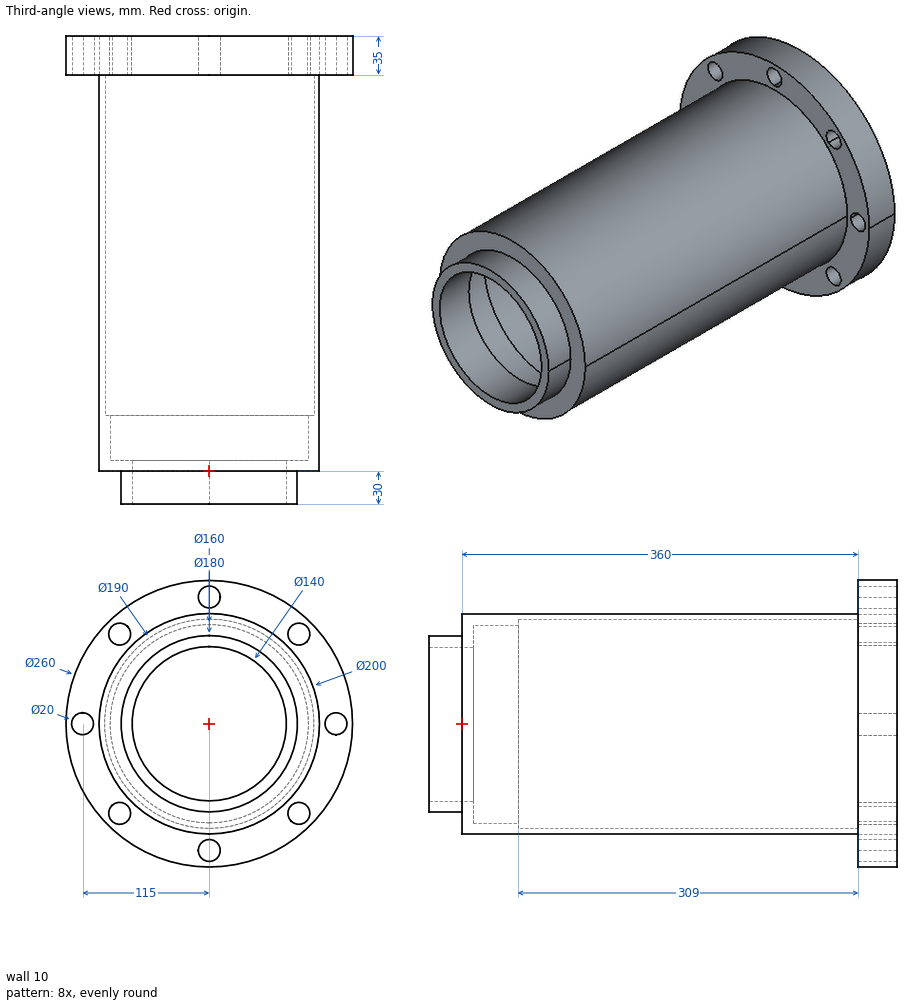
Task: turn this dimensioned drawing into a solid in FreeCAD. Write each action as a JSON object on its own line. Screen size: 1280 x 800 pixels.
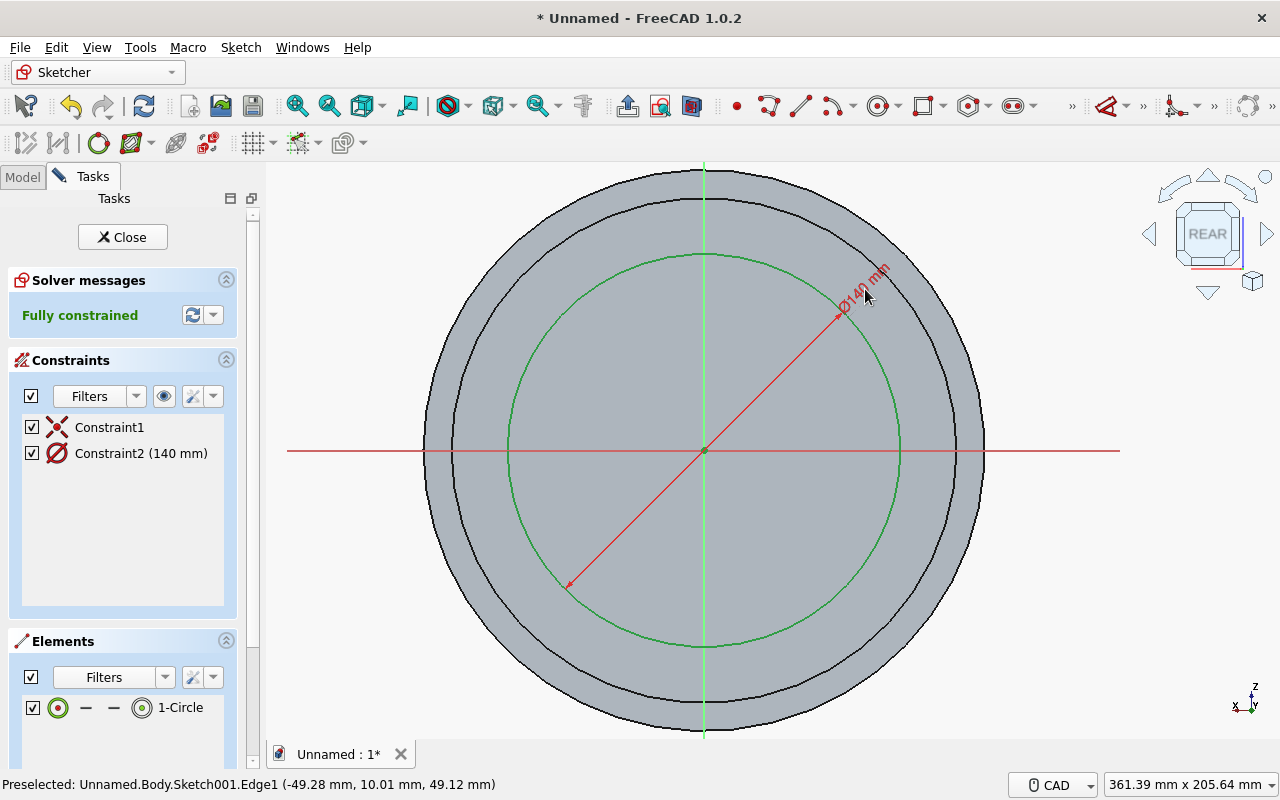
{"action": "left_click", "coordinate": [123, 237]}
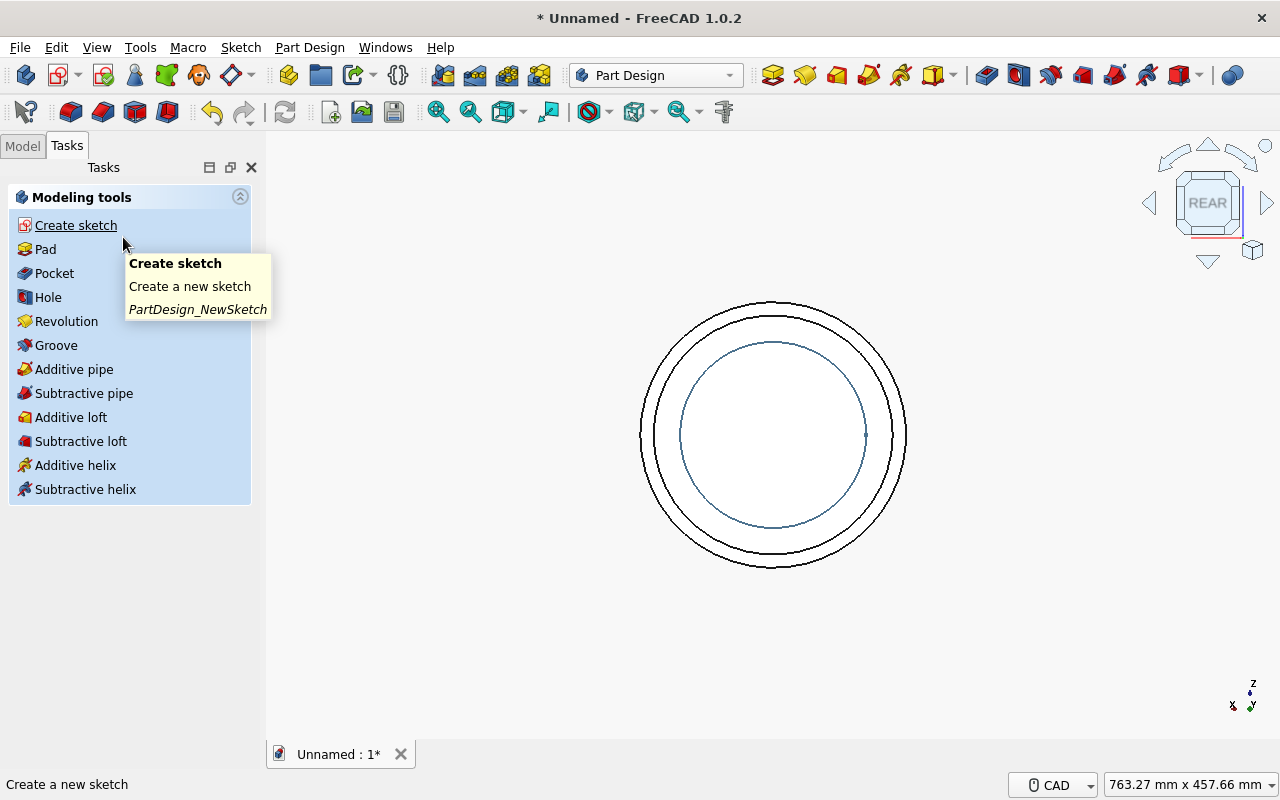
{"action": "left_click", "coordinate": [988, 76]}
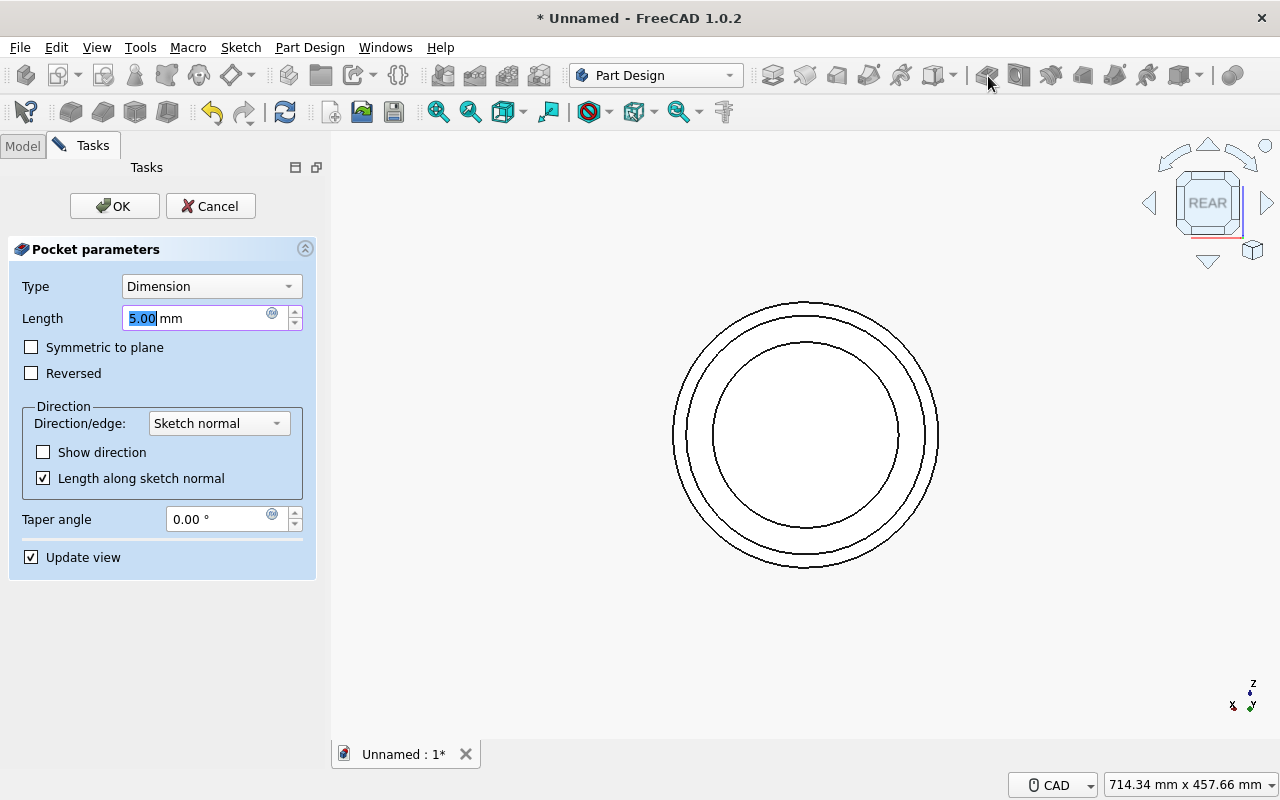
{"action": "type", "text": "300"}
{"action": "key", "text": "Tab"}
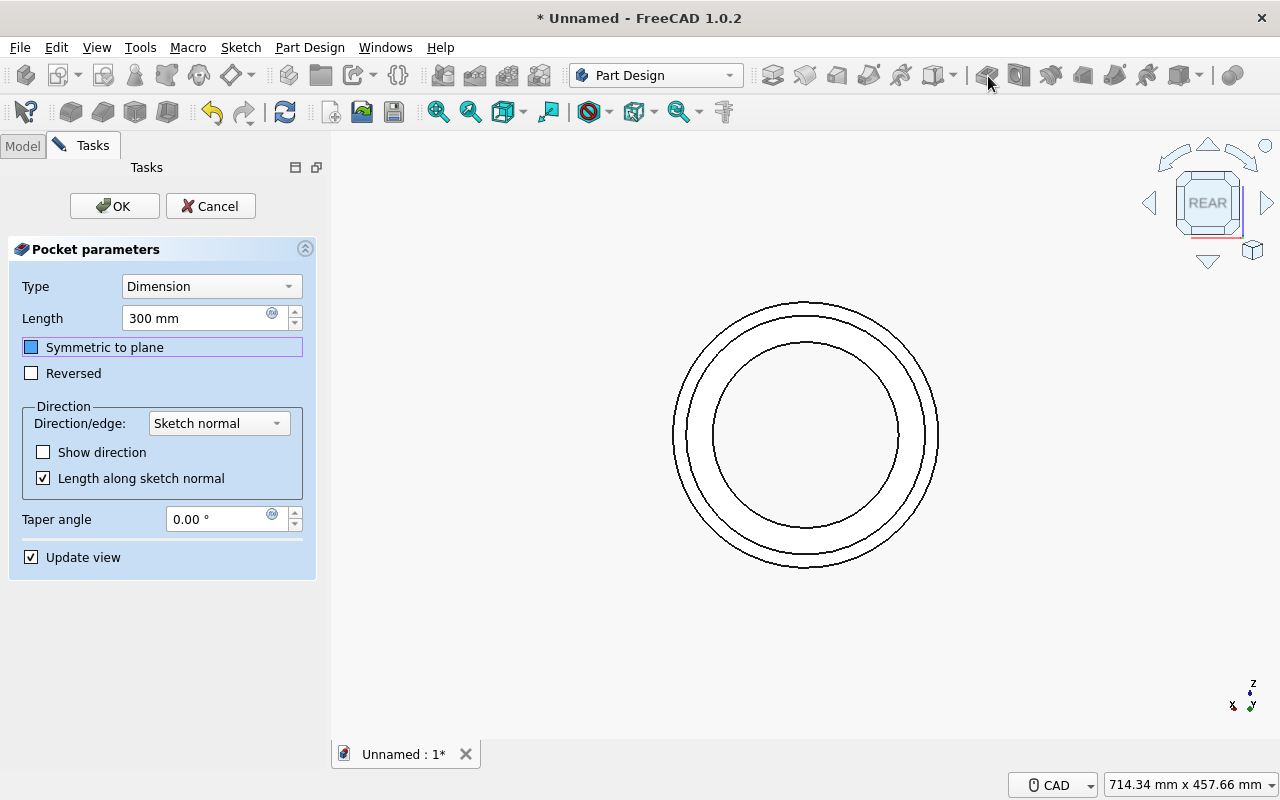
{"action": "left_click", "coordinate": [115, 206]}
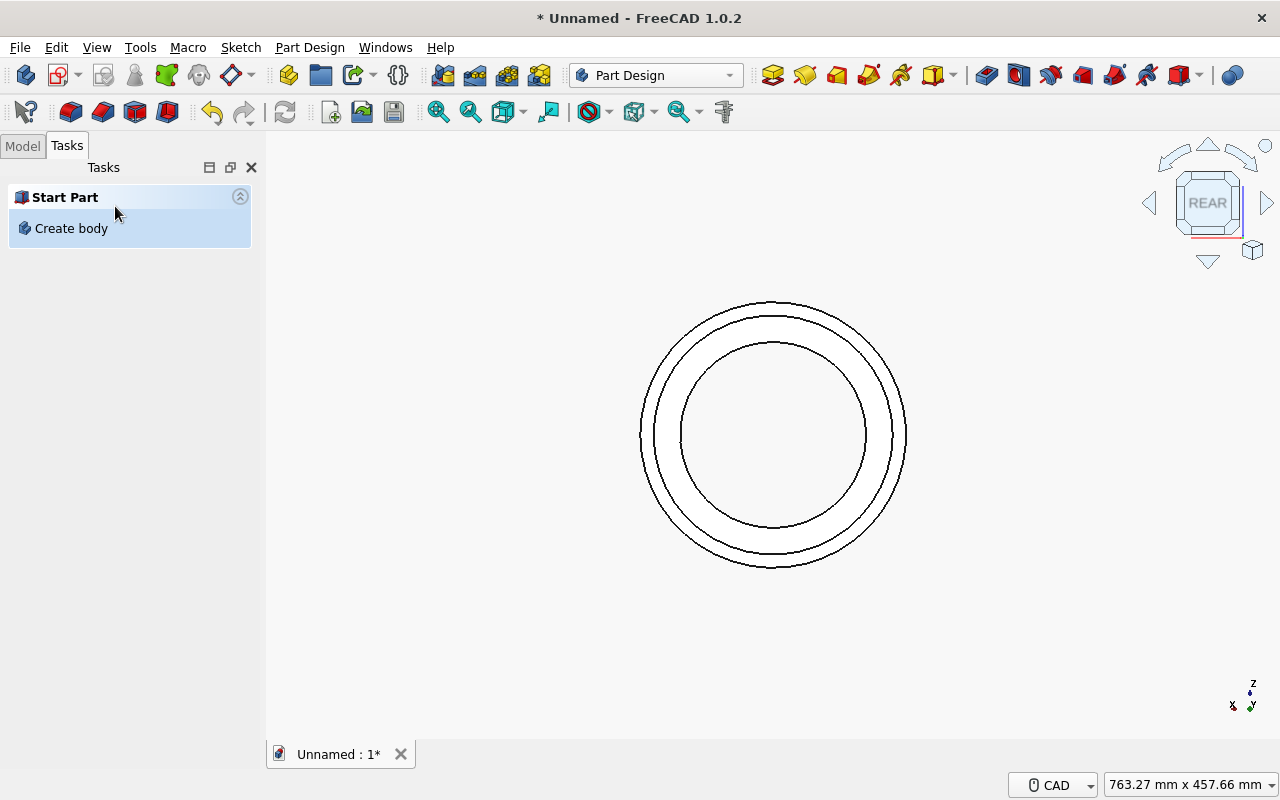
{"action": "left_click", "coordinate": [440, 112]}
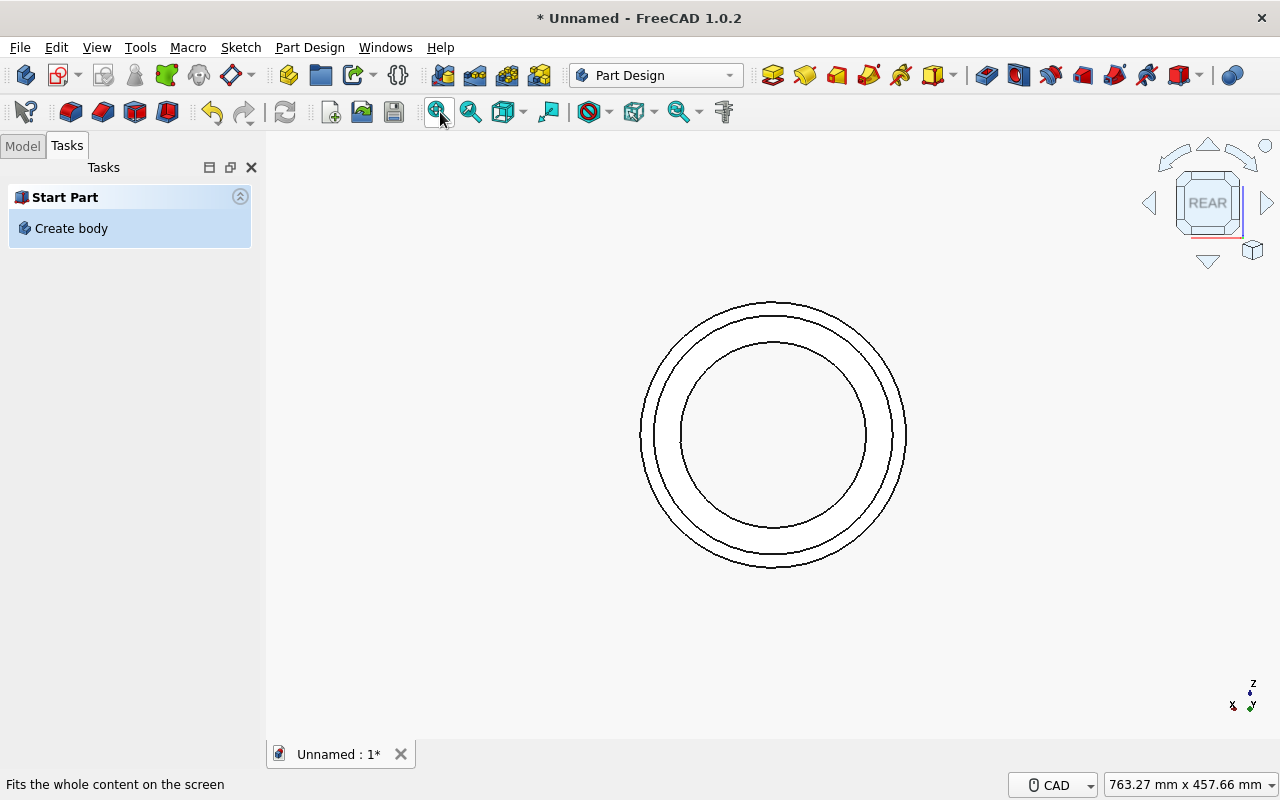
{"action": "left_click", "coordinate": [58, 76]}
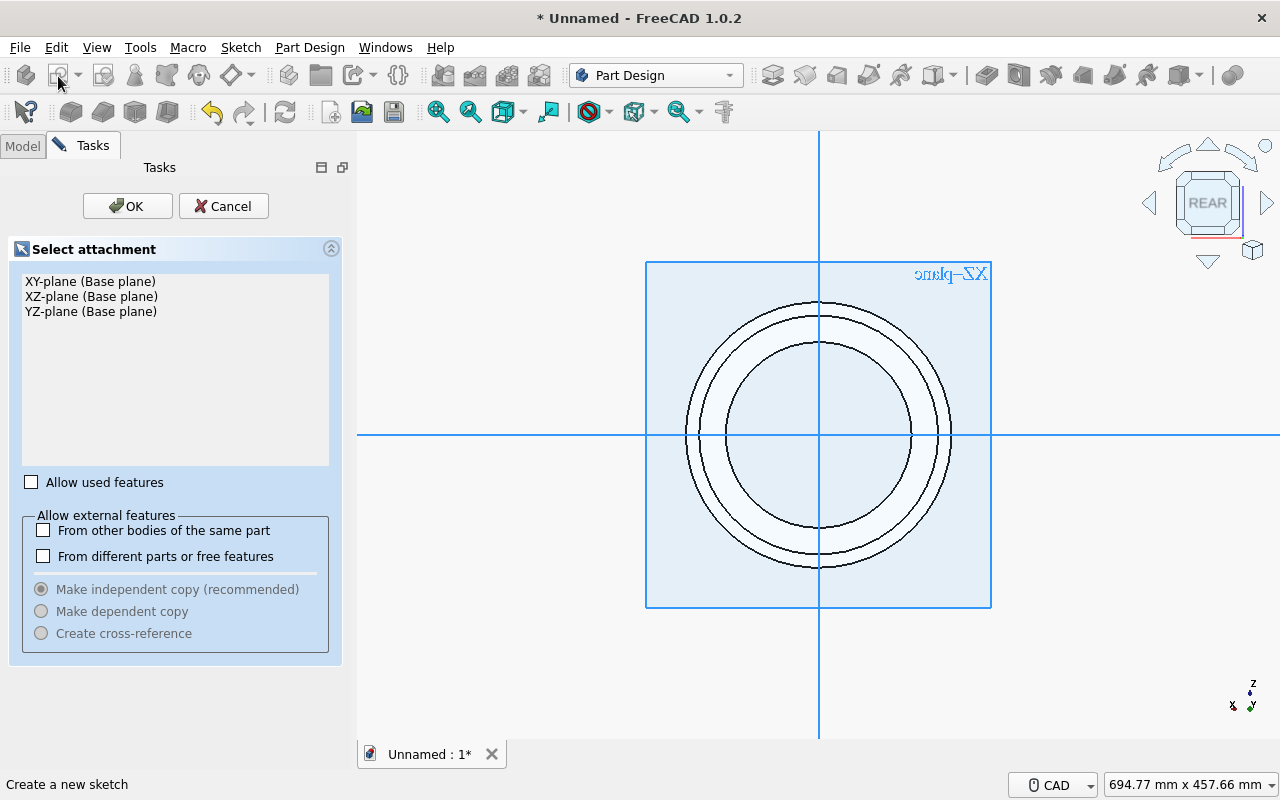
{"action": "left_click", "coordinate": [82, 296]}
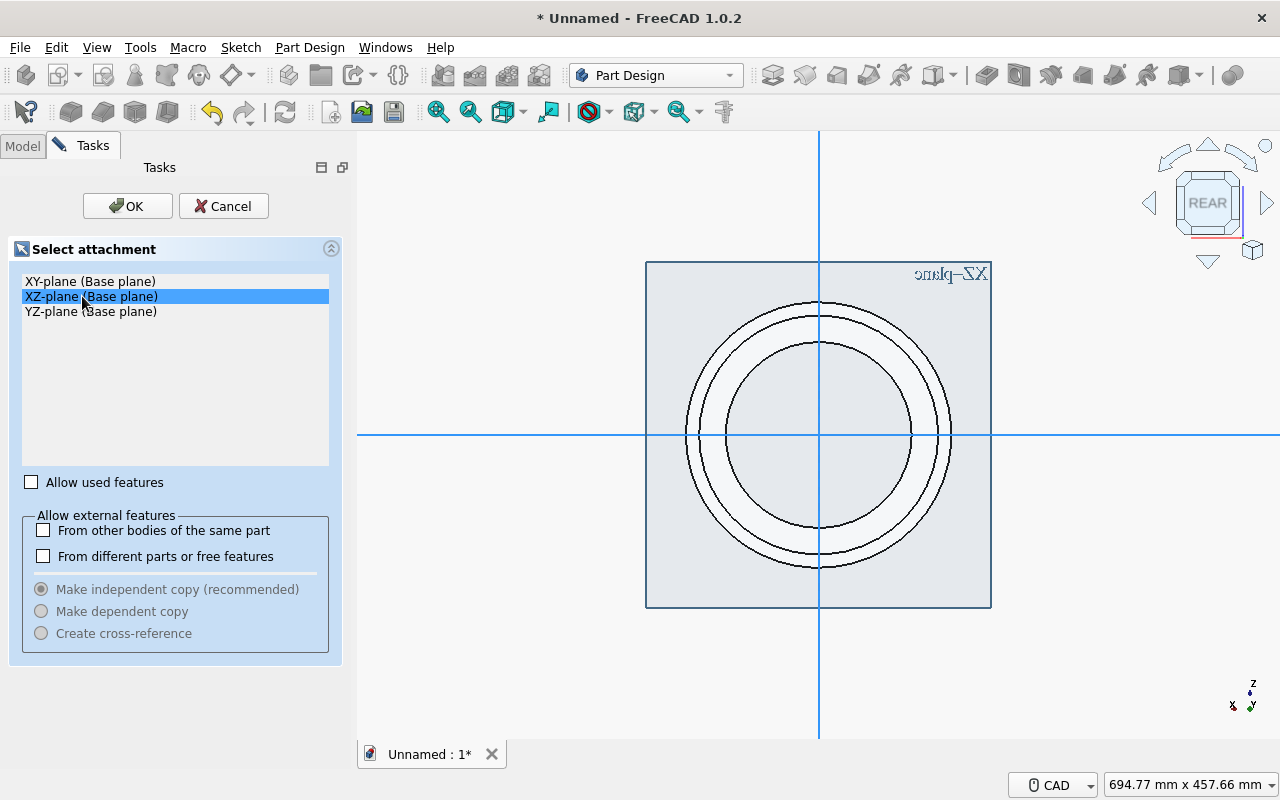
{"action": "left_click", "coordinate": [128, 206]}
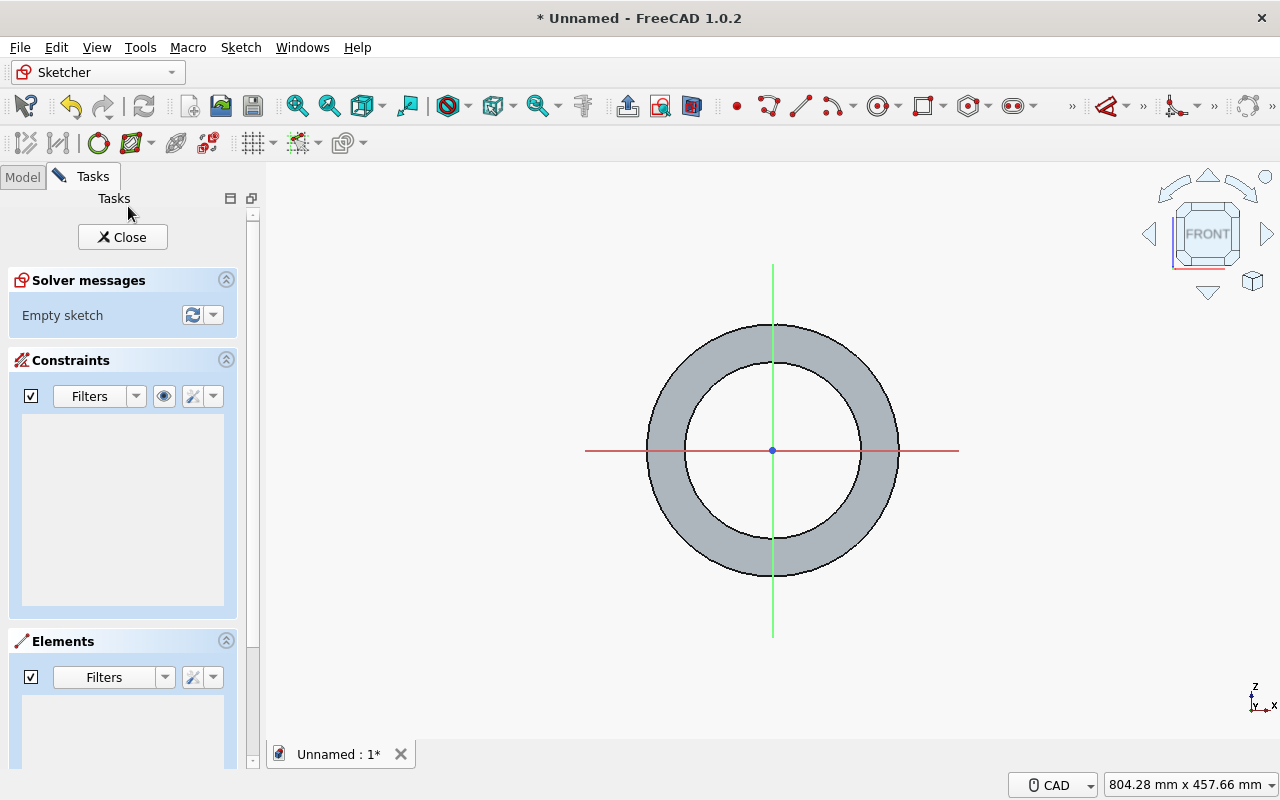
{"action": "scroll", "coordinate": [856, 450], "scroll_direction": "up", "scroll_amount": 3}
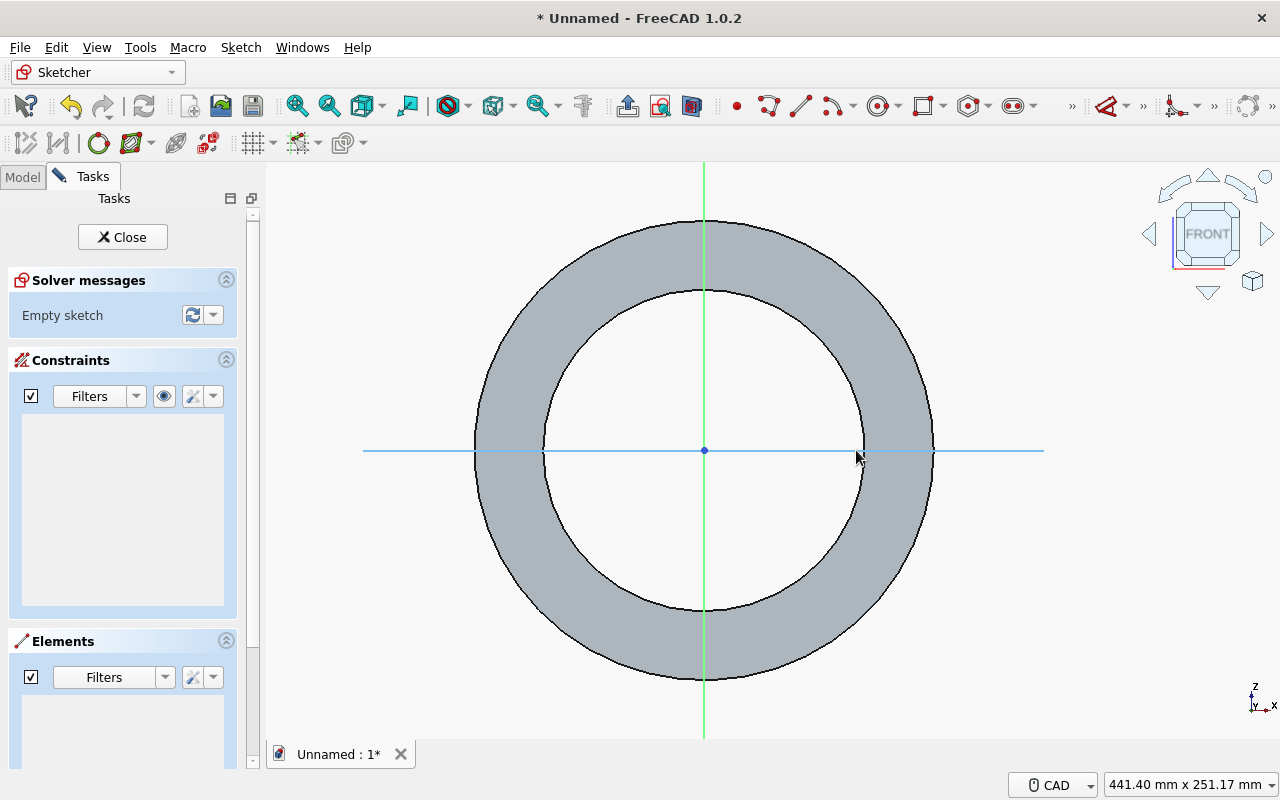
{"action": "left_click", "coordinate": [878, 106]}